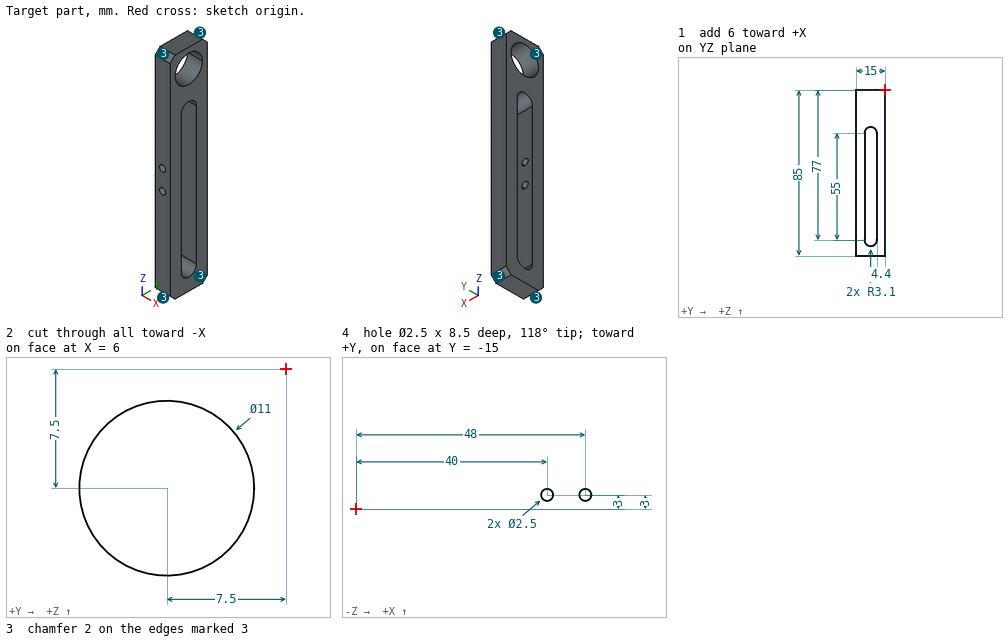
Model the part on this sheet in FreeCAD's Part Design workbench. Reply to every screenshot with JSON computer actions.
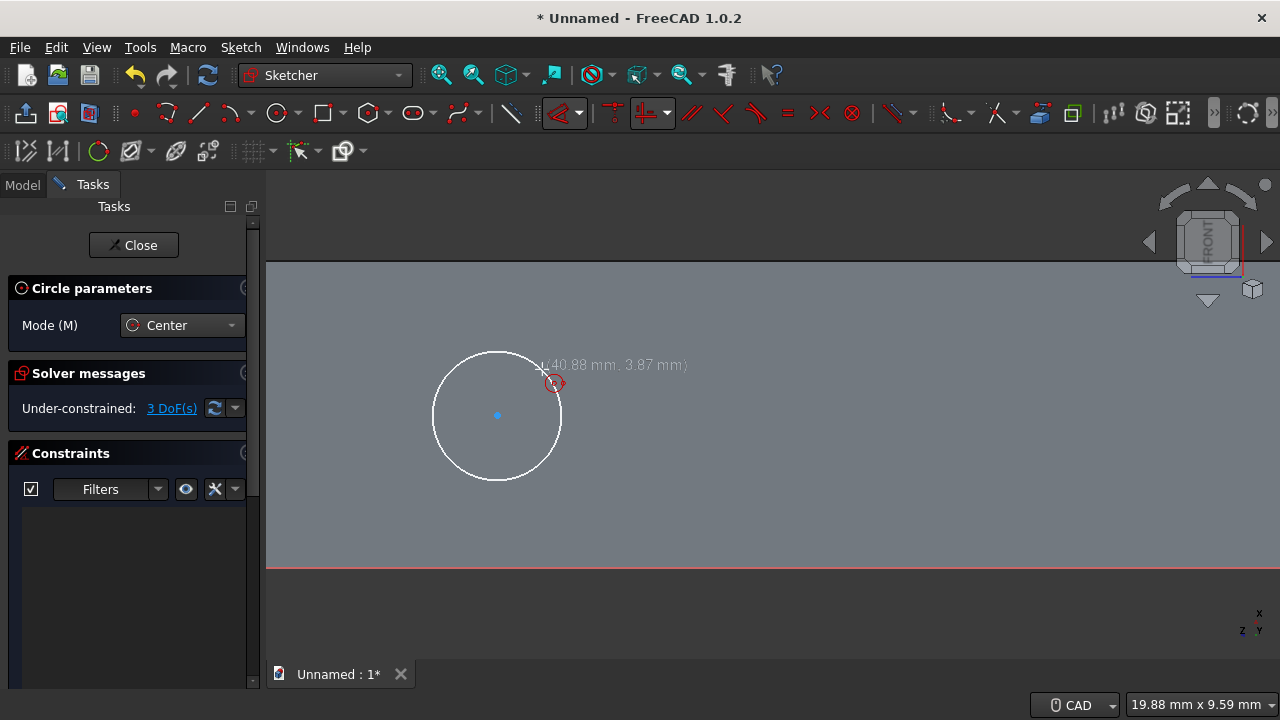
{"action": "left_click", "coordinate": [905, 415]}
{"action": "left_click", "coordinate": [950, 369]}
{"action": "key", "text": "Escape"}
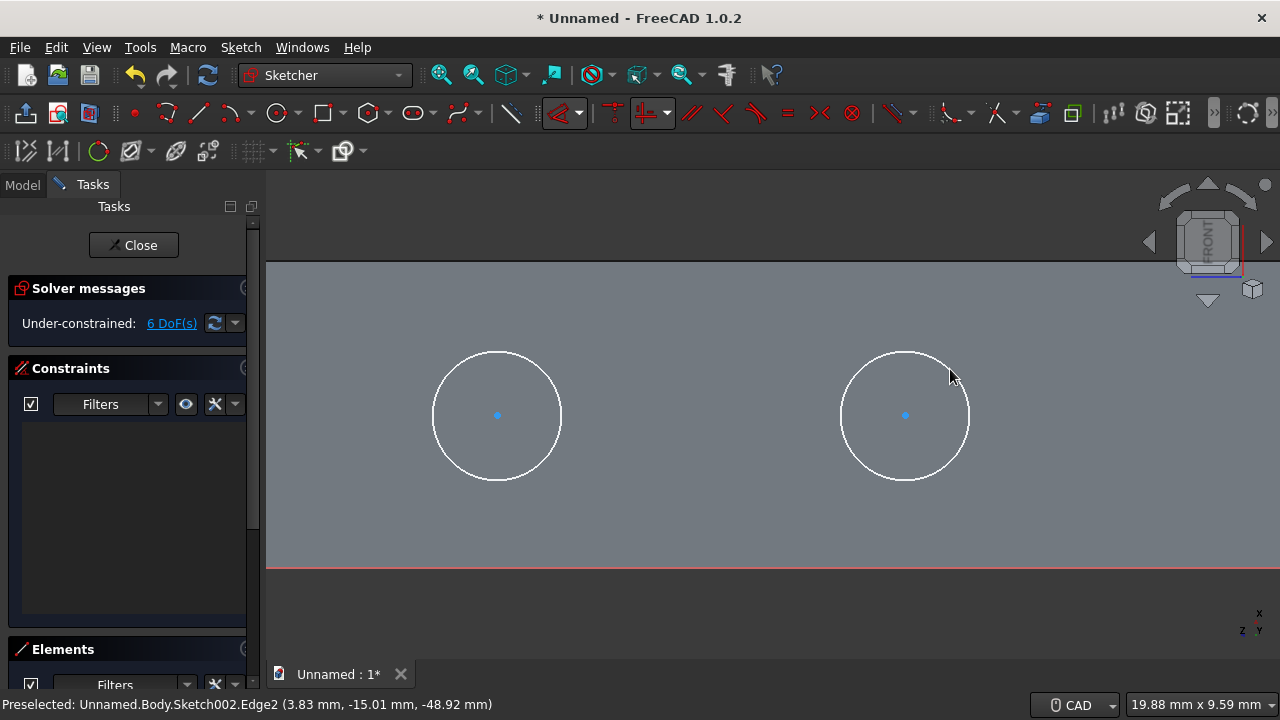
{"action": "left_click", "coordinate": [542, 370]}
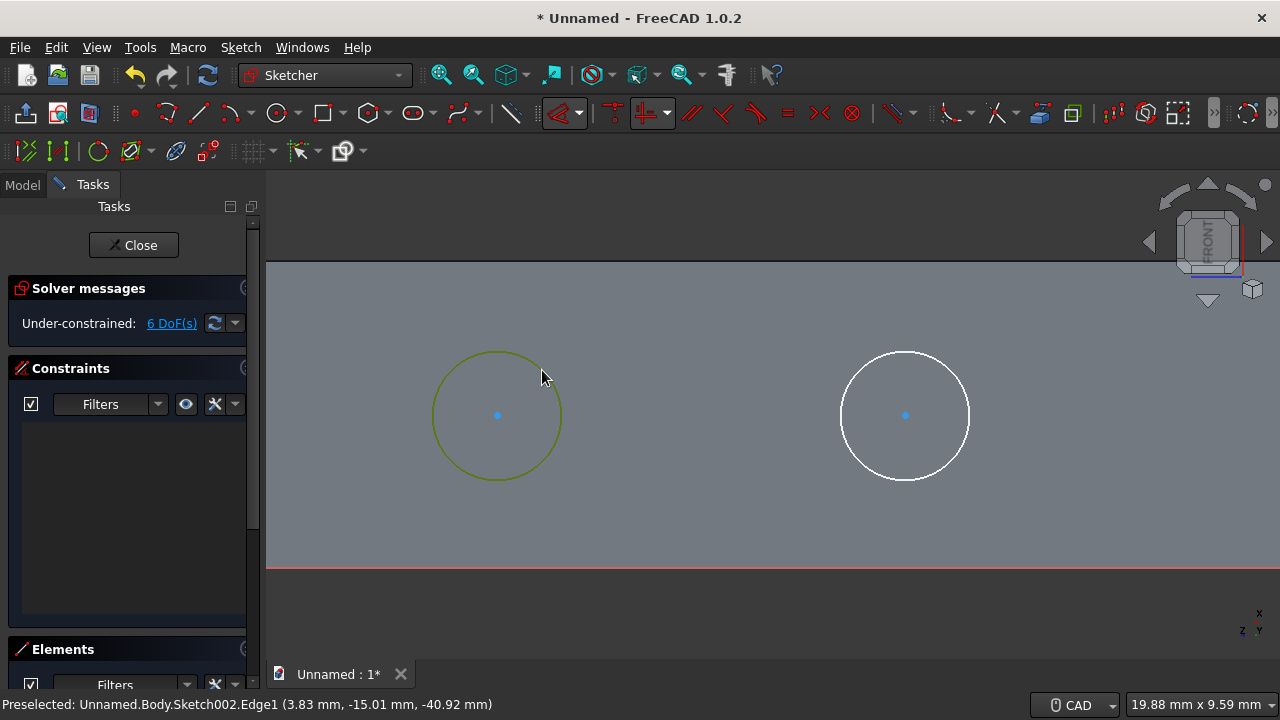
{"action": "left_click", "coordinate": [950, 370]}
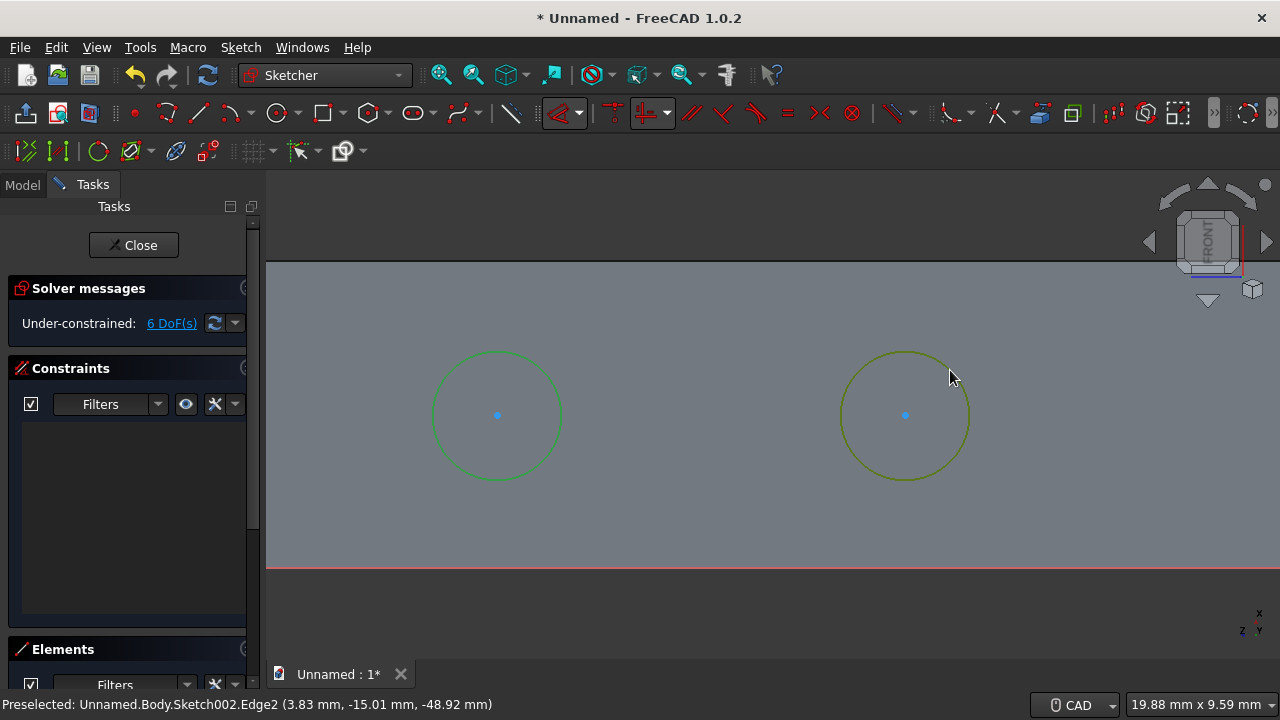
{"action": "left_click", "coordinate": [788, 114]}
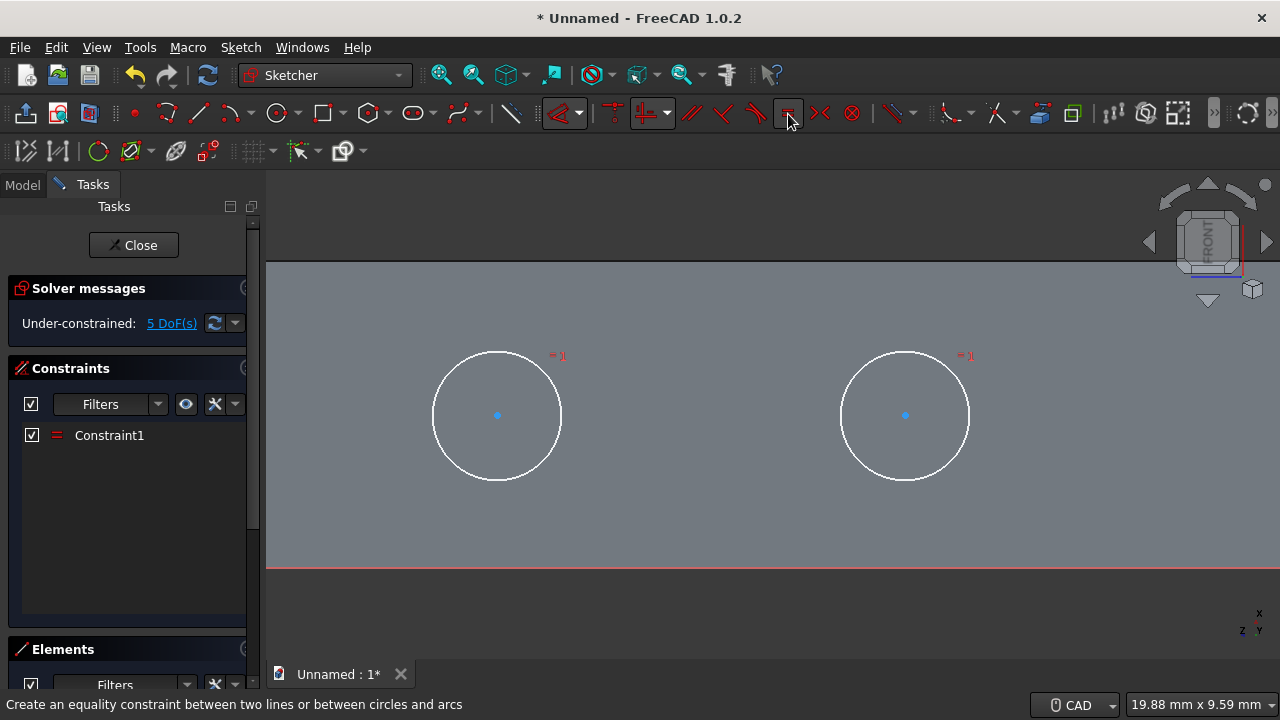
{"action": "left_click", "coordinate": [558, 114]}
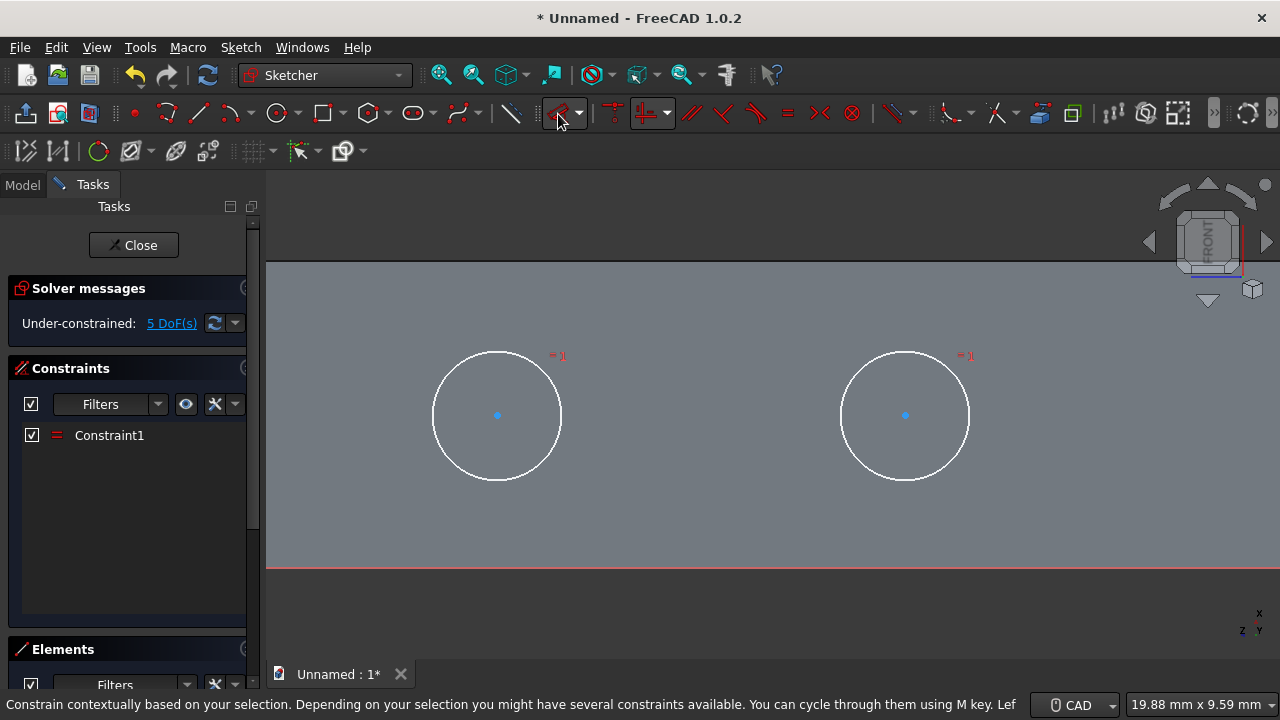
{"action": "left_click", "coordinate": [542, 370]}
{"action": "left_click", "coordinate": [564, 347]}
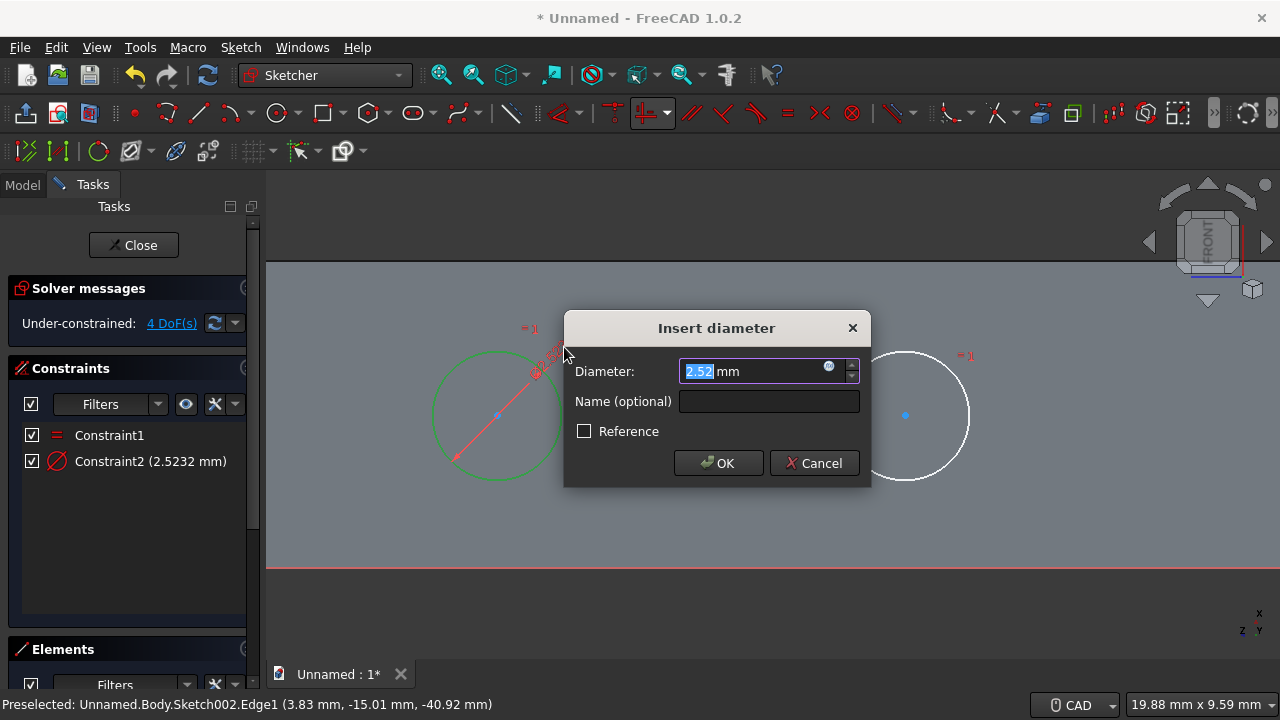
{"action": "type", "text": "2.5"}
{"action": "key", "text": "Return"}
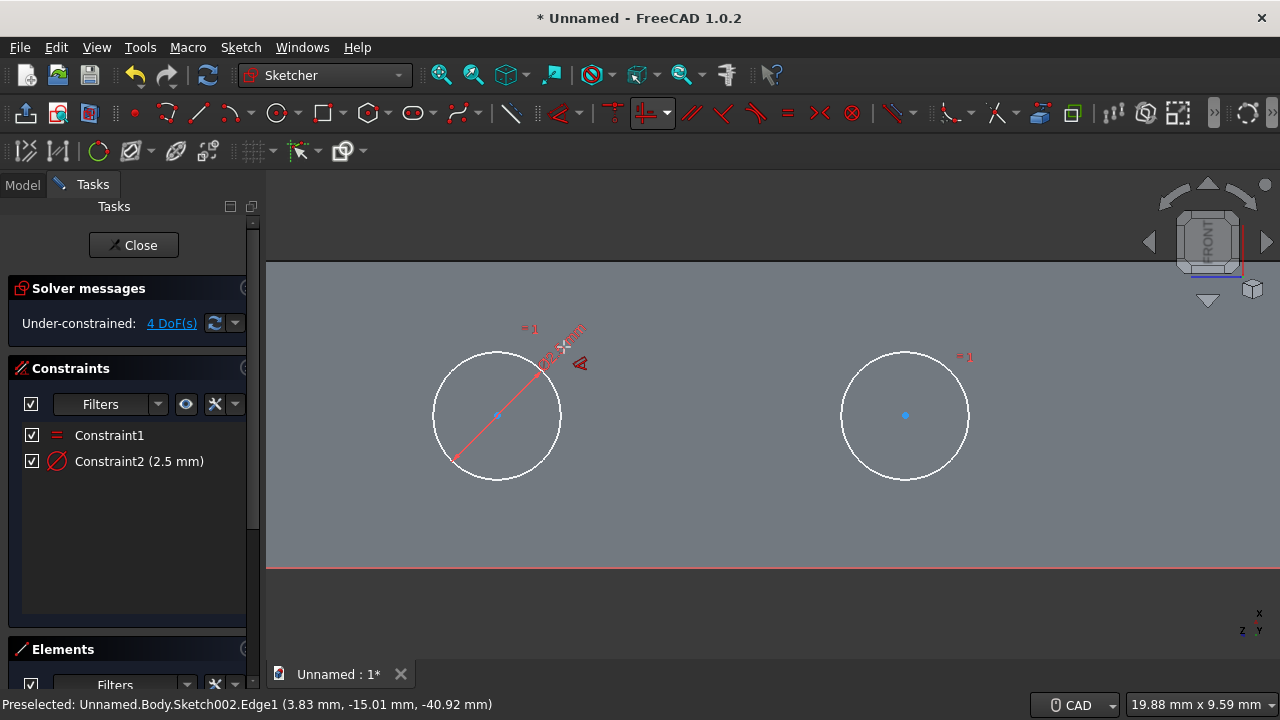
{"action": "left_click", "coordinate": [497, 416]}
{"action": "left_click", "coordinate": [531, 492]}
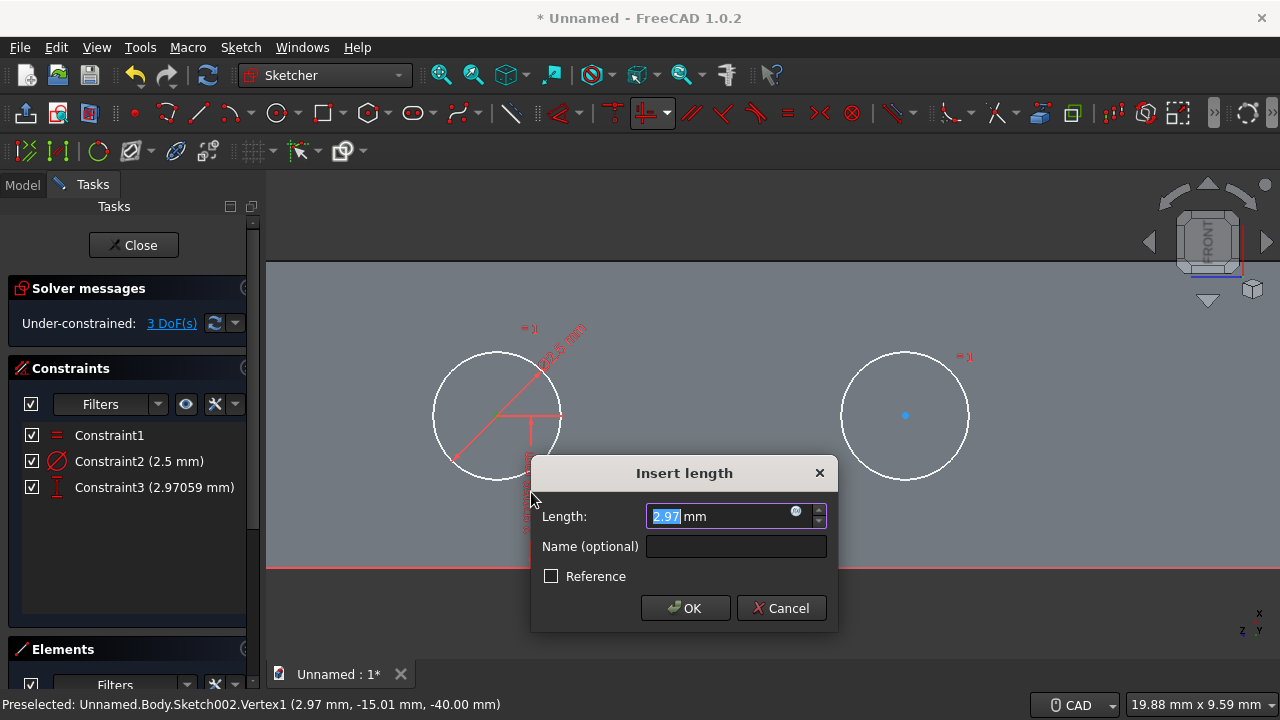
{"action": "type", "text": "3"}
{"action": "key", "text": "Return"}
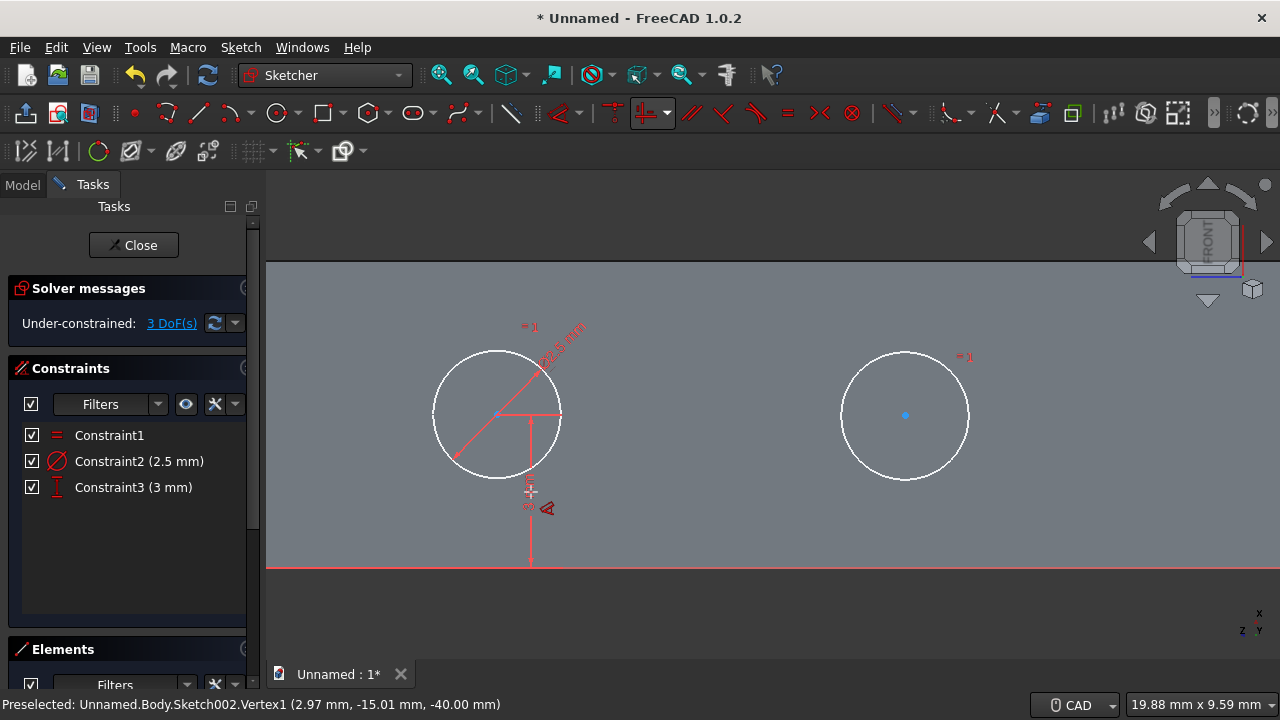
{"action": "left_click", "coordinate": [905, 416]}
{"action": "left_click", "coordinate": [939, 492]}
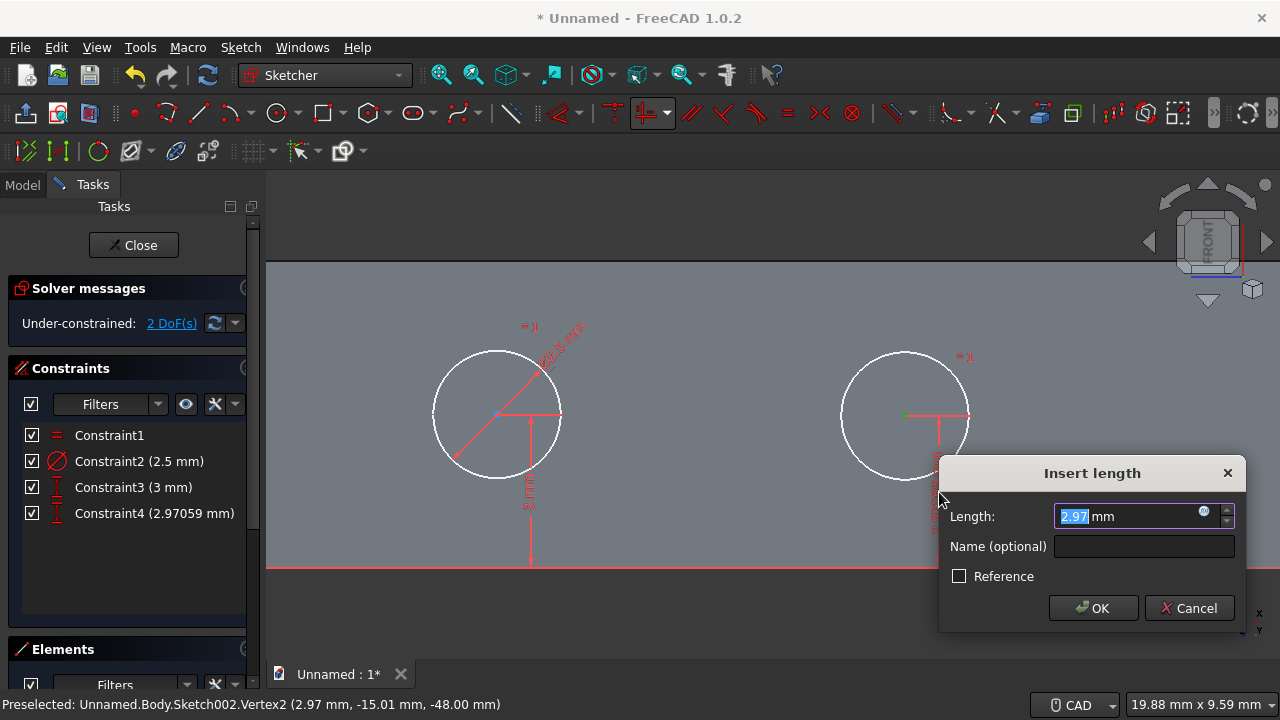
{"action": "type", "text": "3"}
{"action": "key", "text": "Return"}